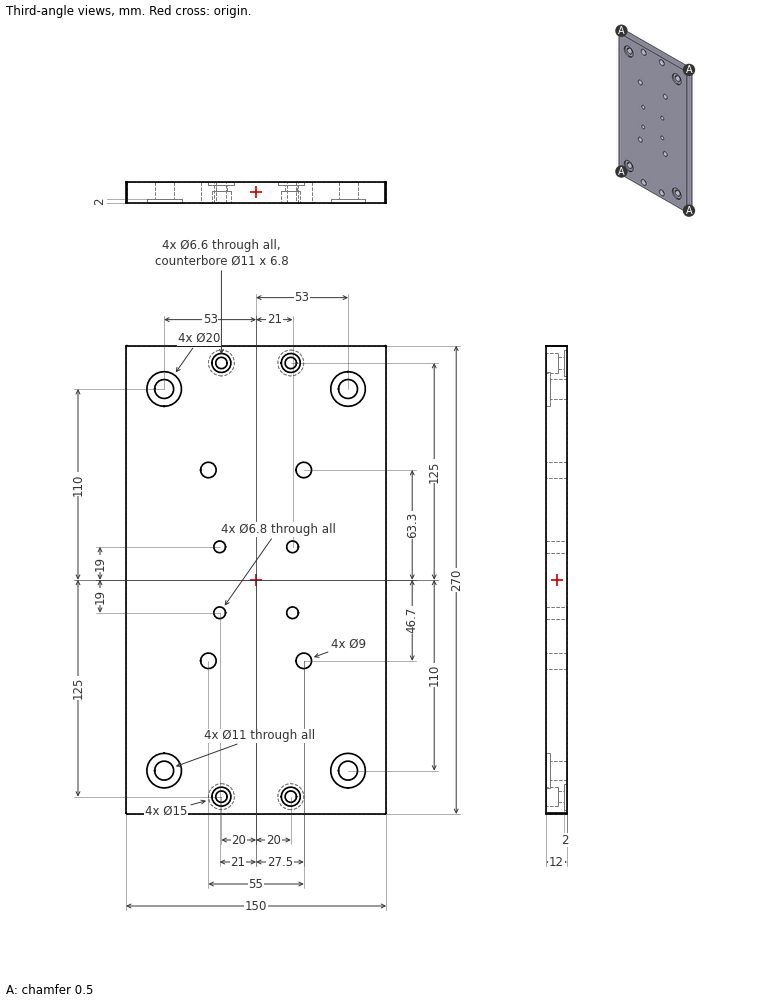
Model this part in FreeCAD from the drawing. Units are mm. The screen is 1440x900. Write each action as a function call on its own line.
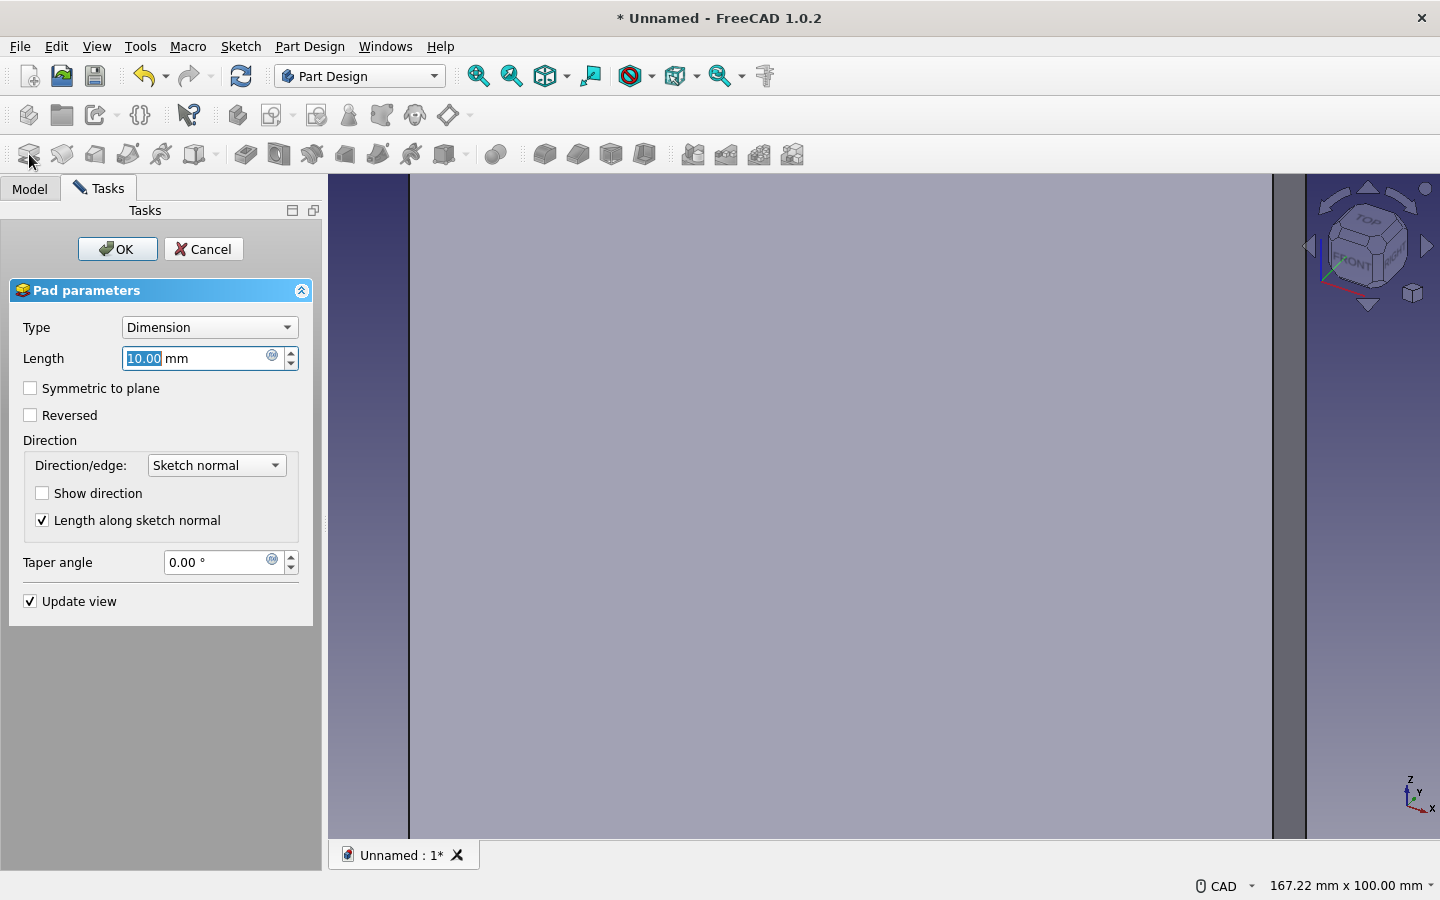
text(12)
key(Tab)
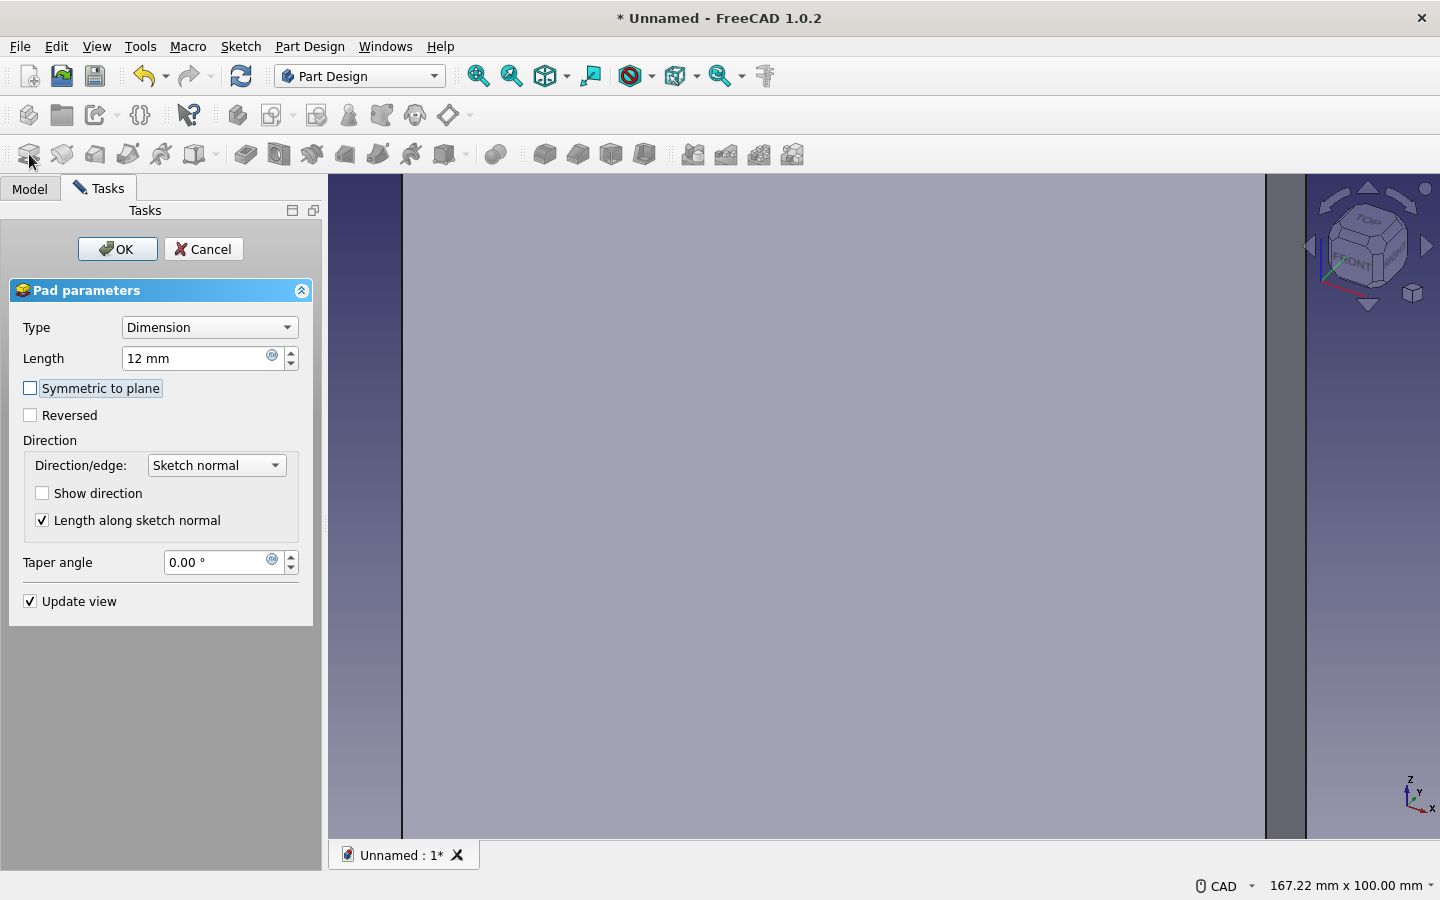
click(31, 388)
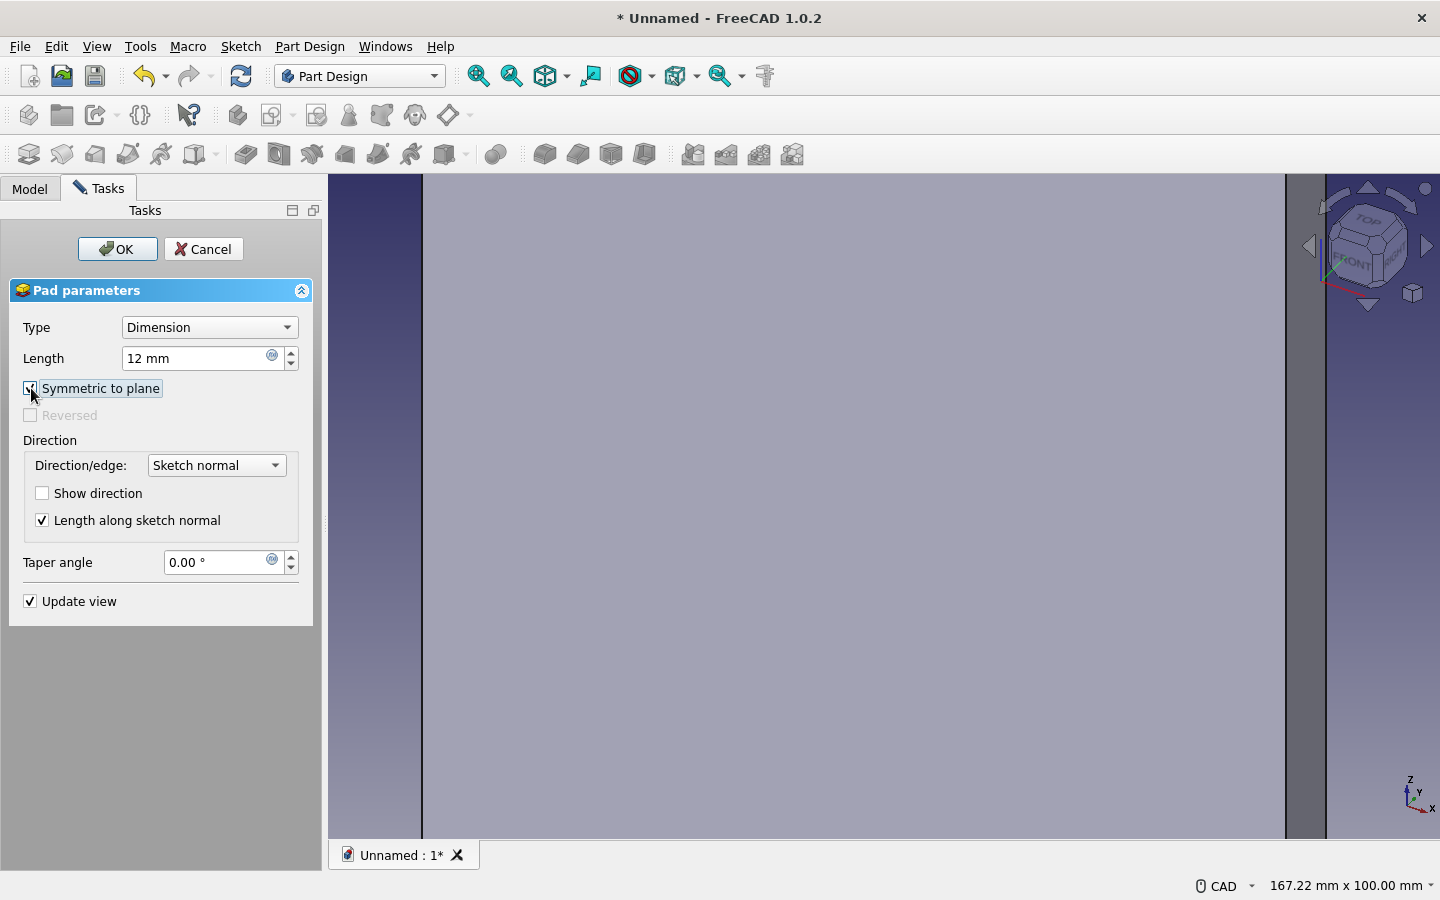
click(118, 249)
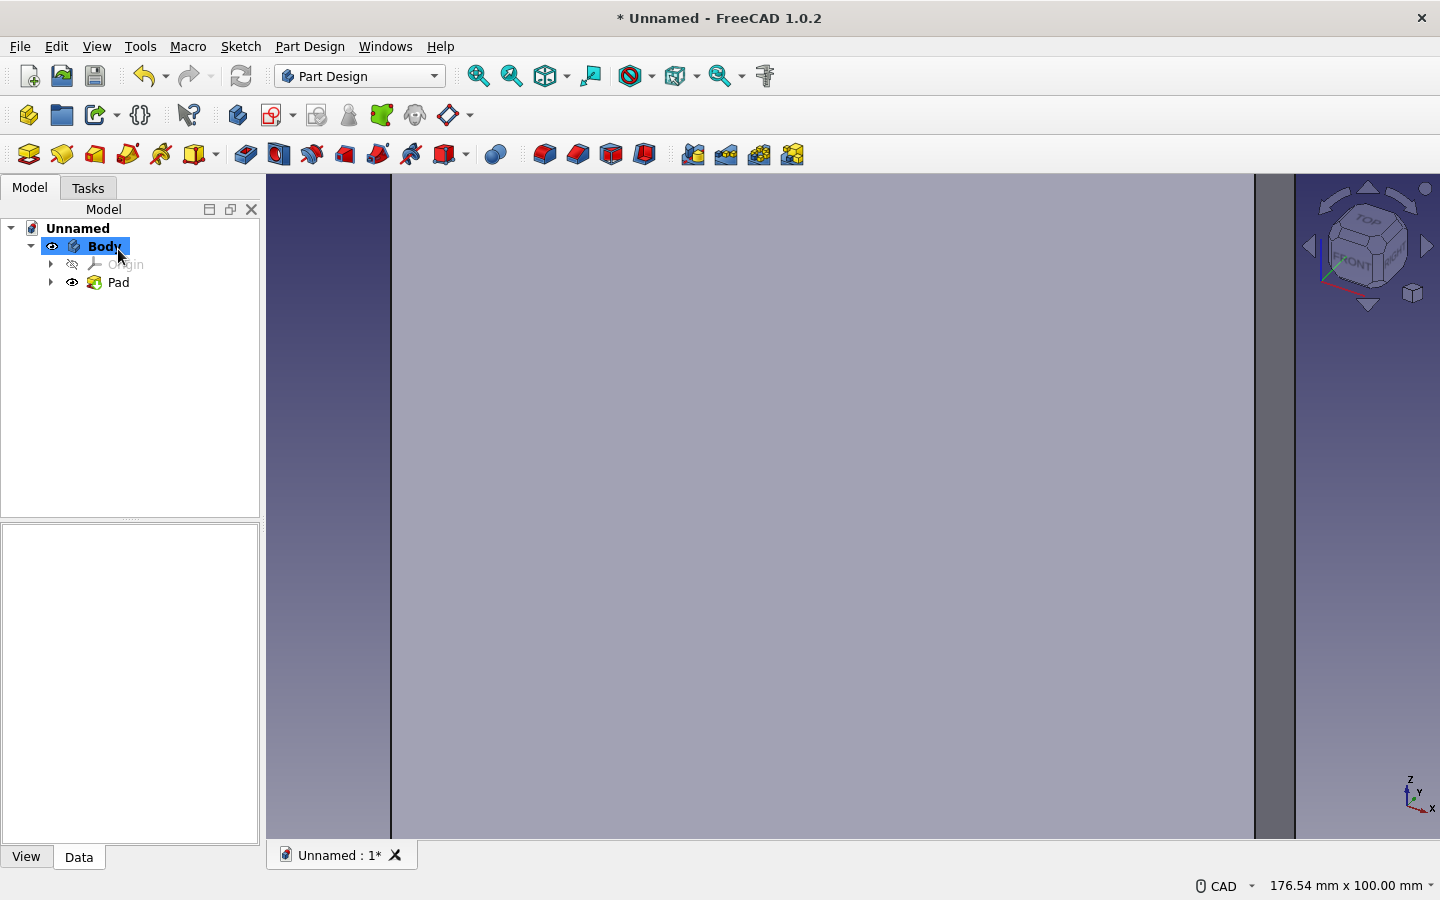
key(v)
key(f)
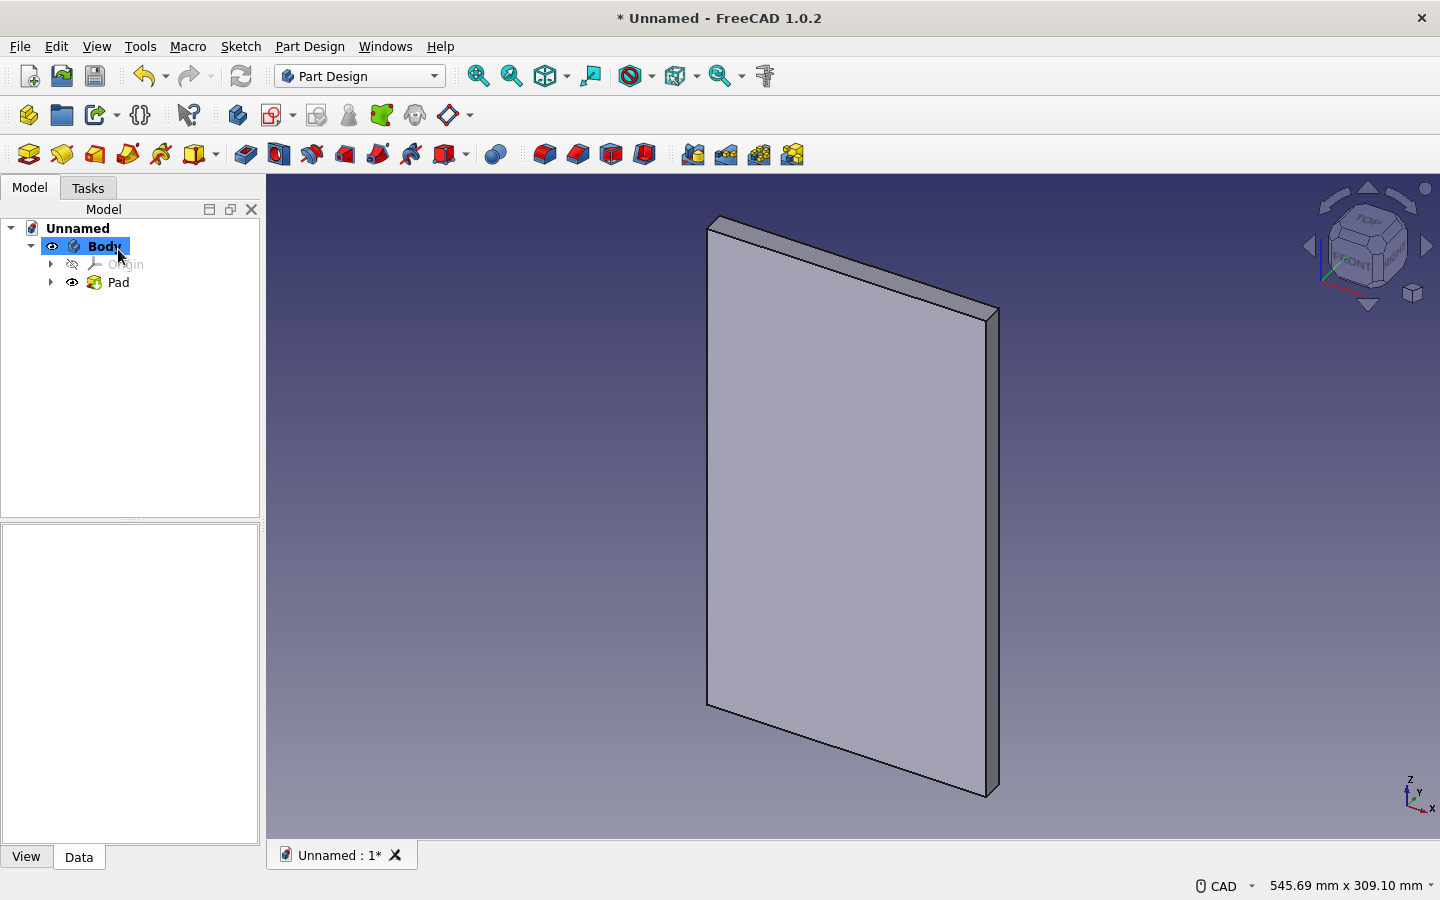
click(847, 444)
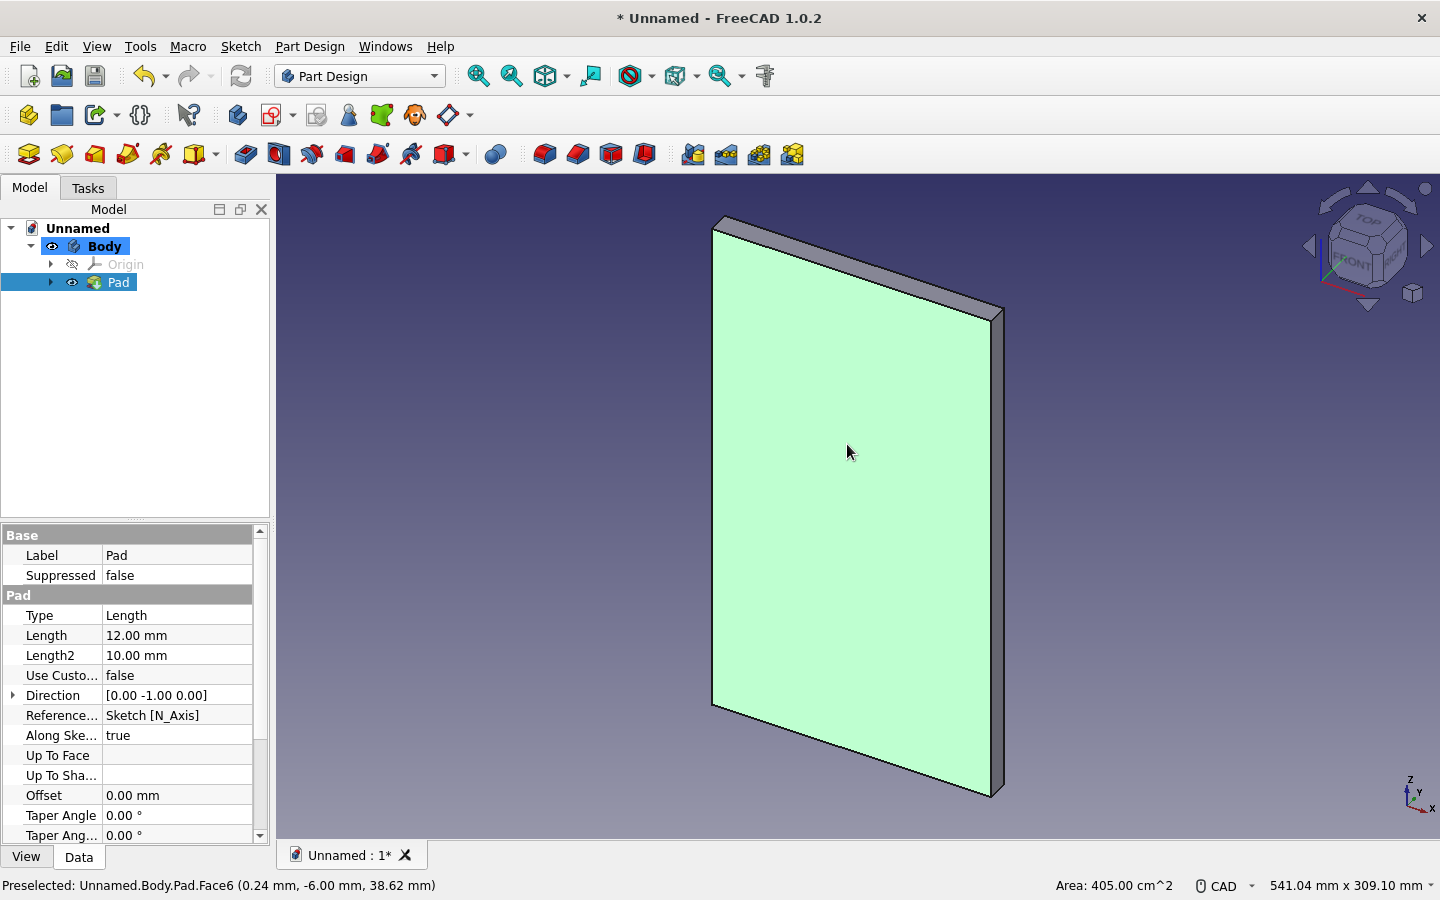
click(270, 116)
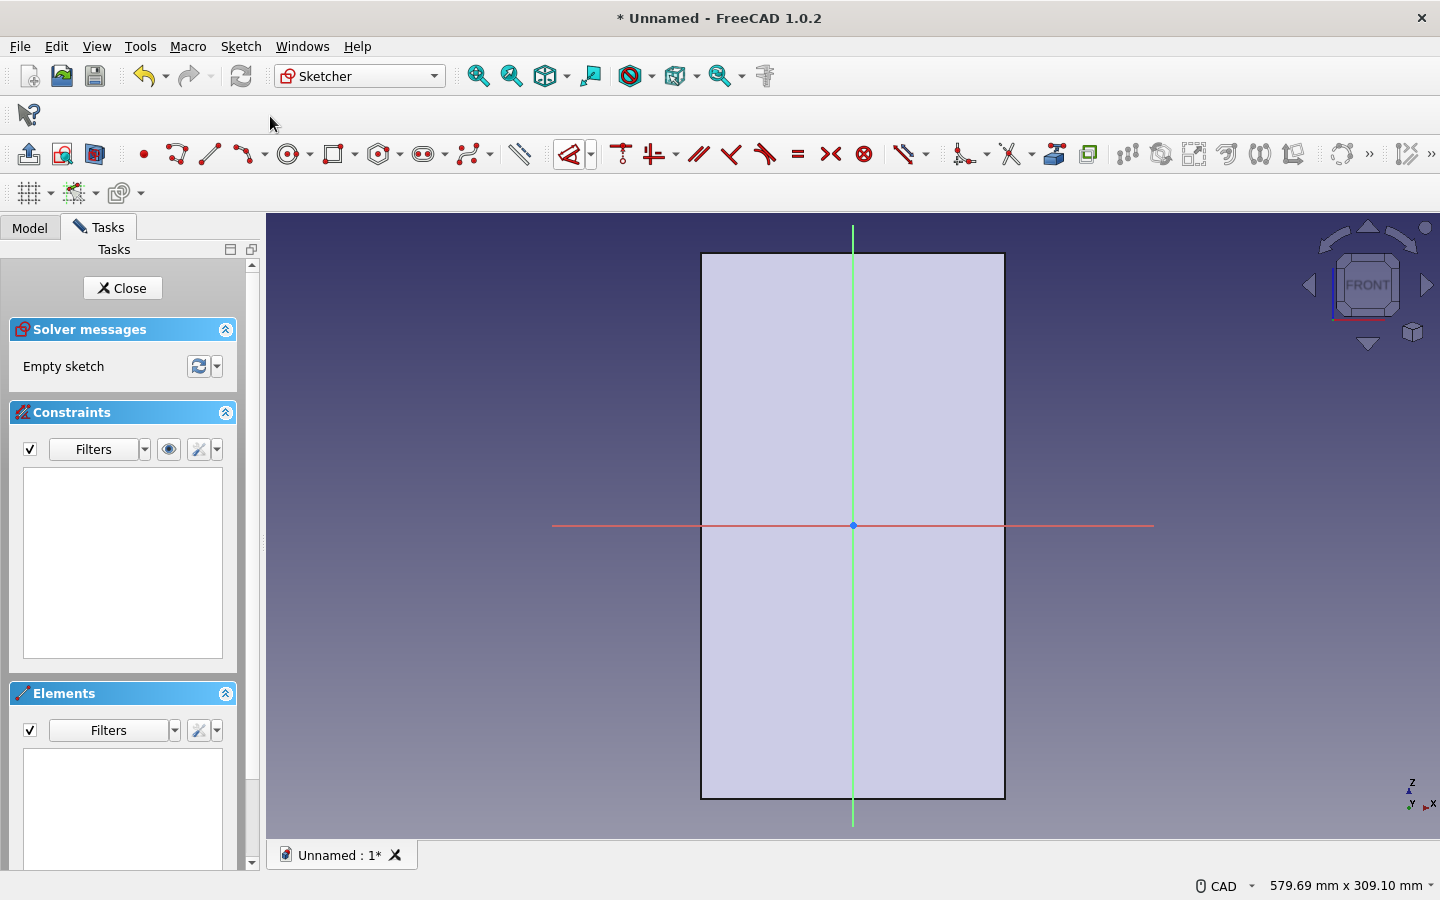
key(g)
key(c)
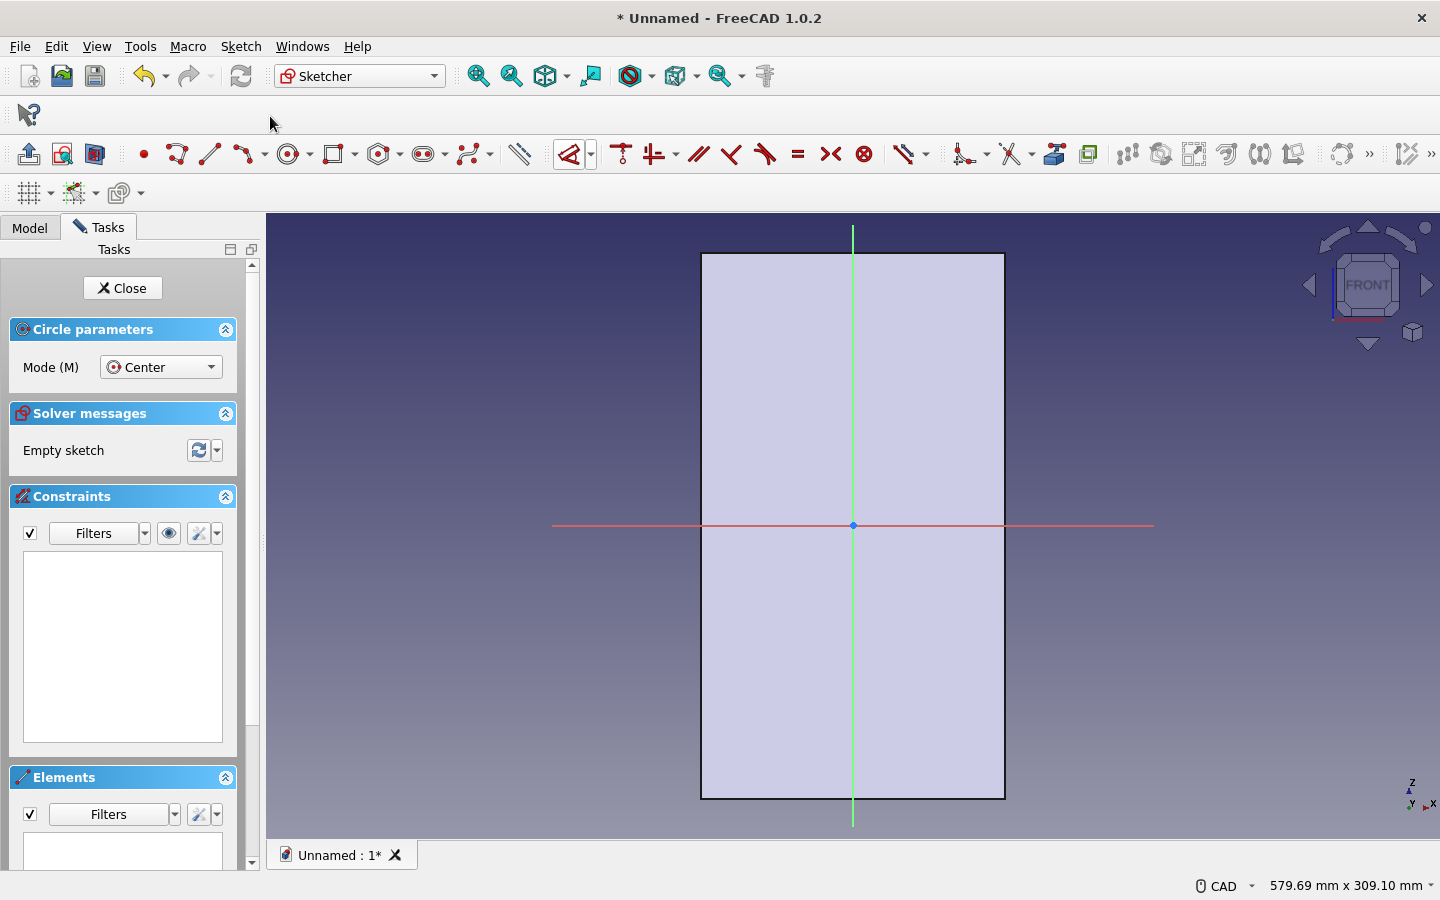
click(746, 303)
click(760, 289)